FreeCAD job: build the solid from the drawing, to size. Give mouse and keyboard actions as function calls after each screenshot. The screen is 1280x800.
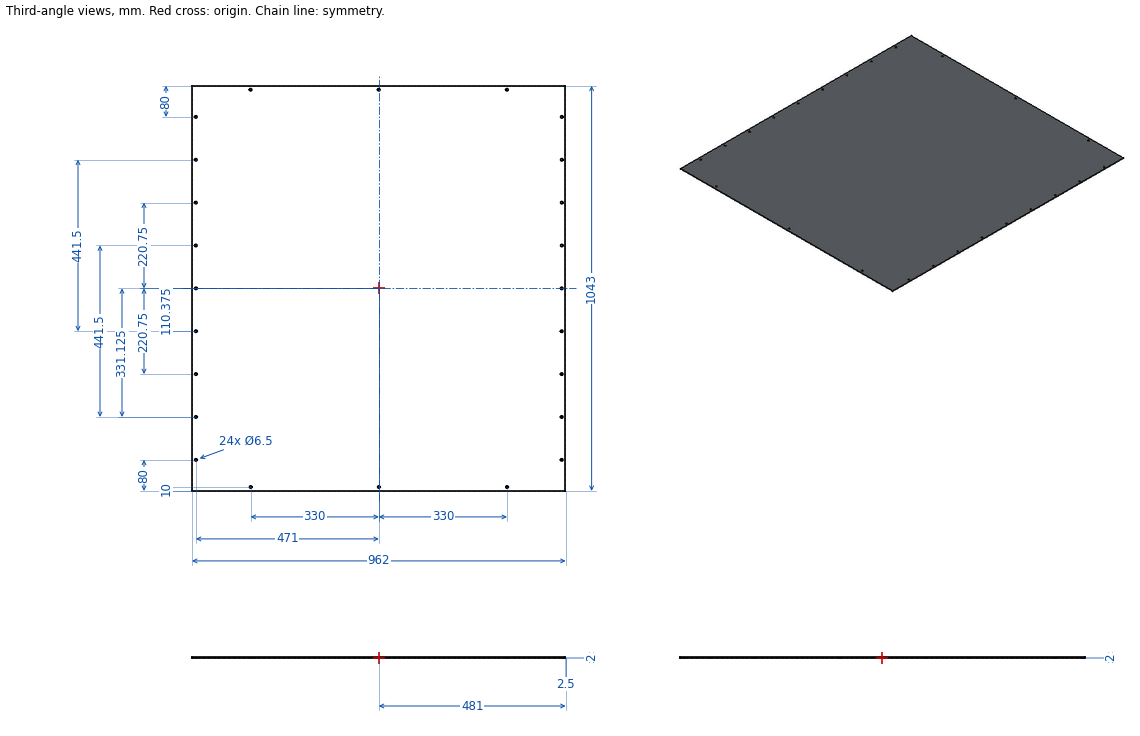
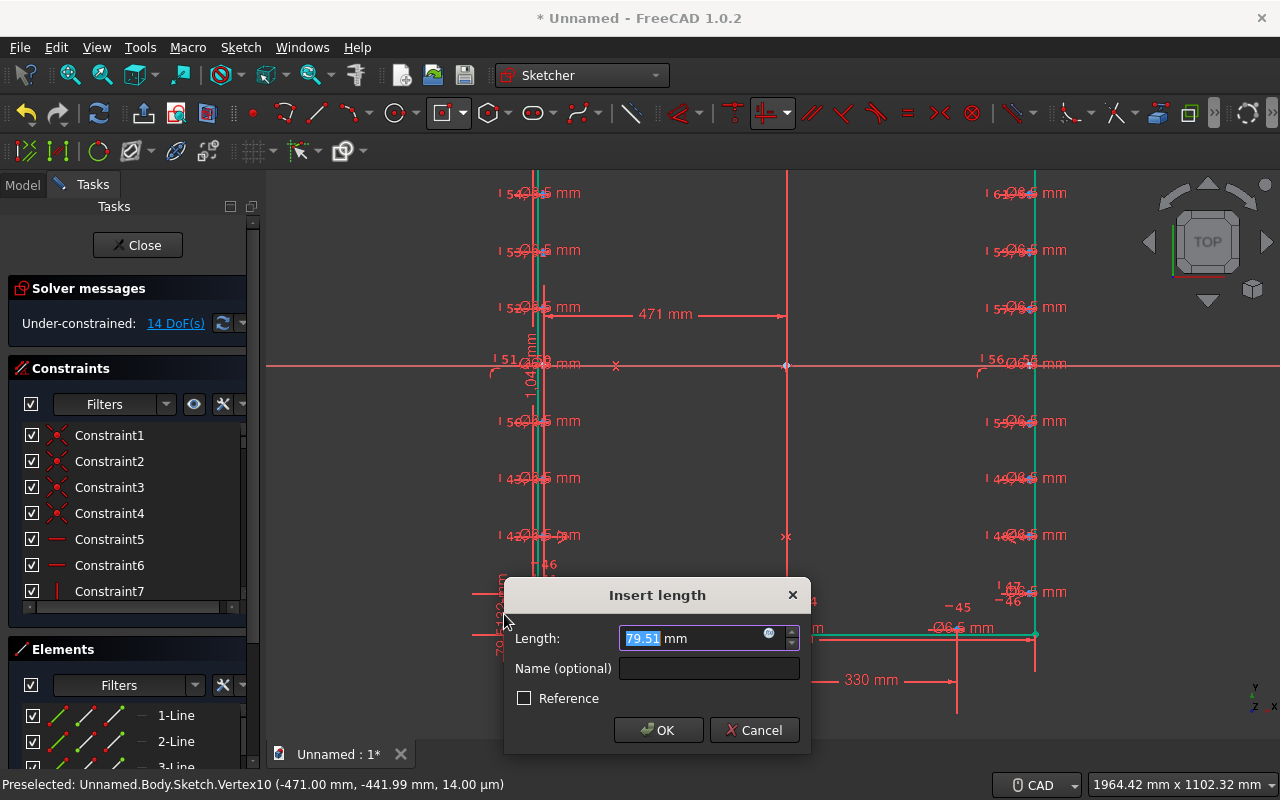
text(80)
key(Return)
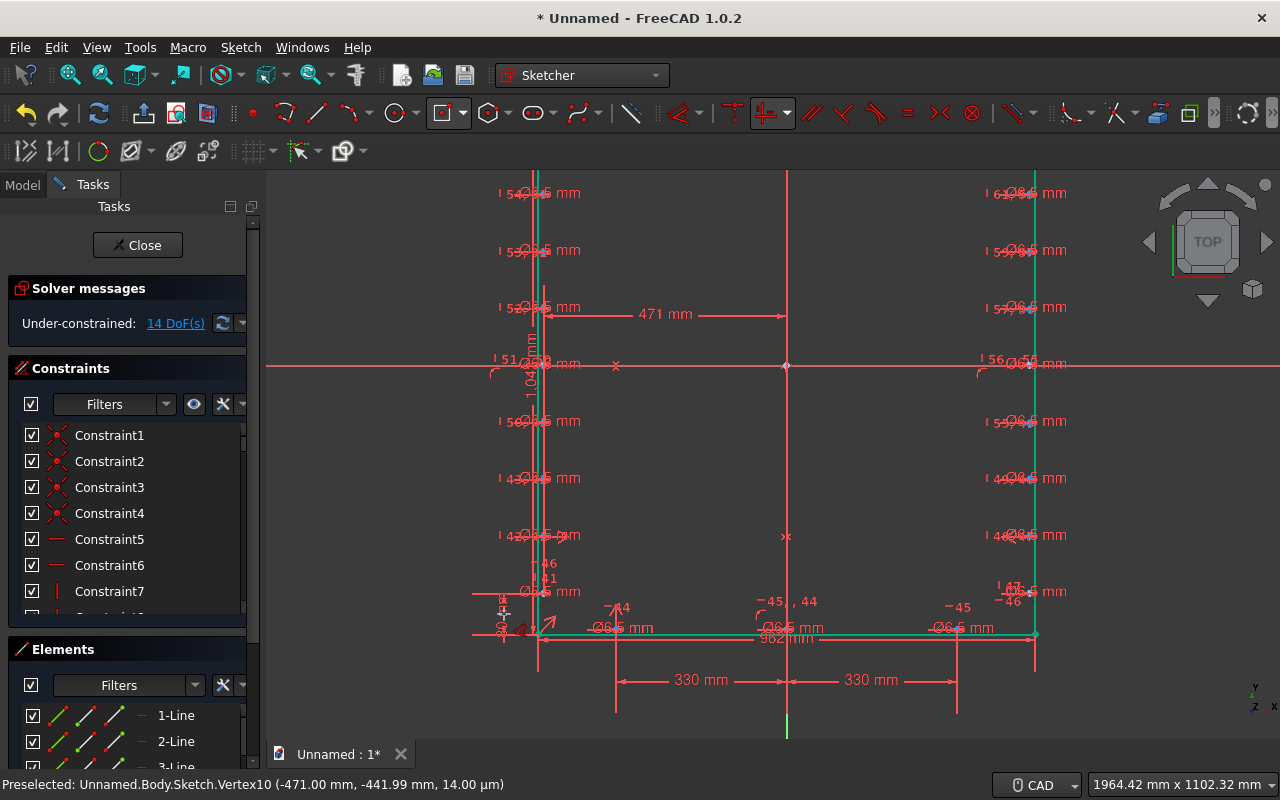
scroll(538, 635, up, 11)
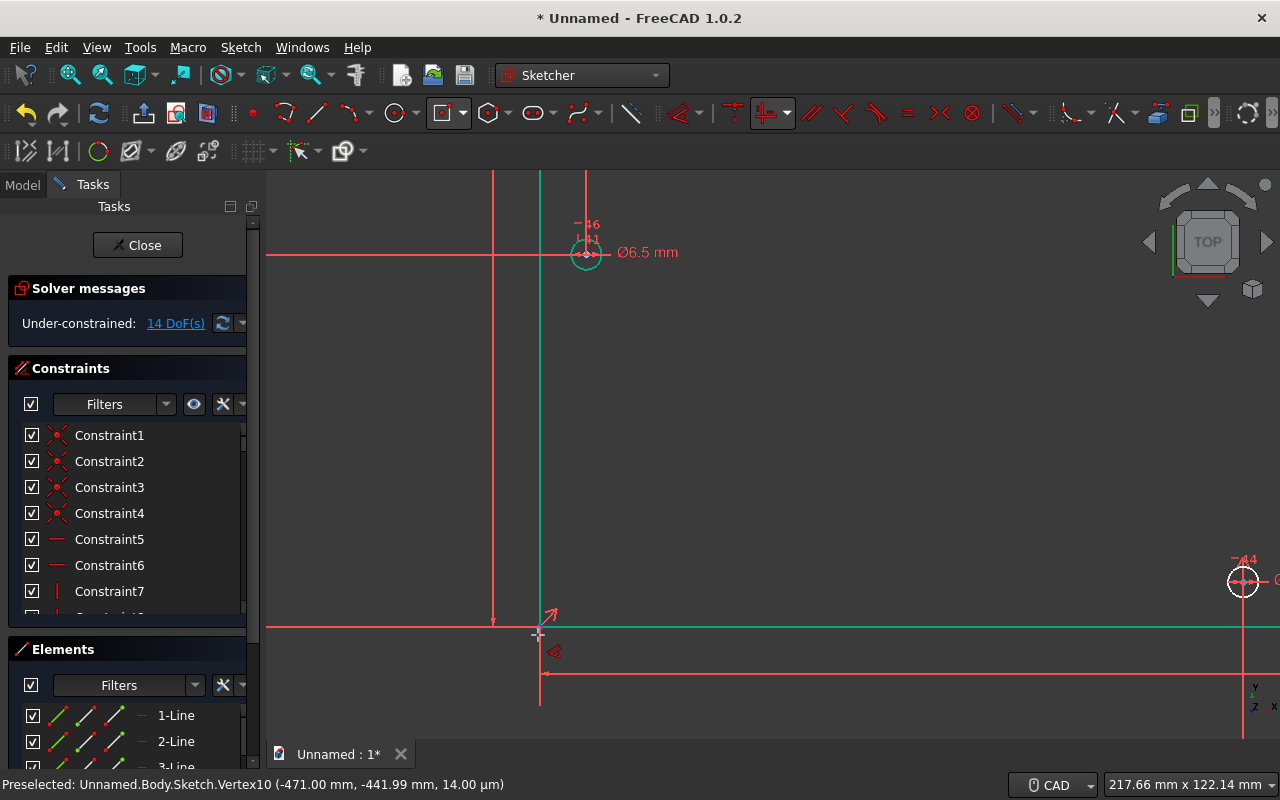
click(540, 627)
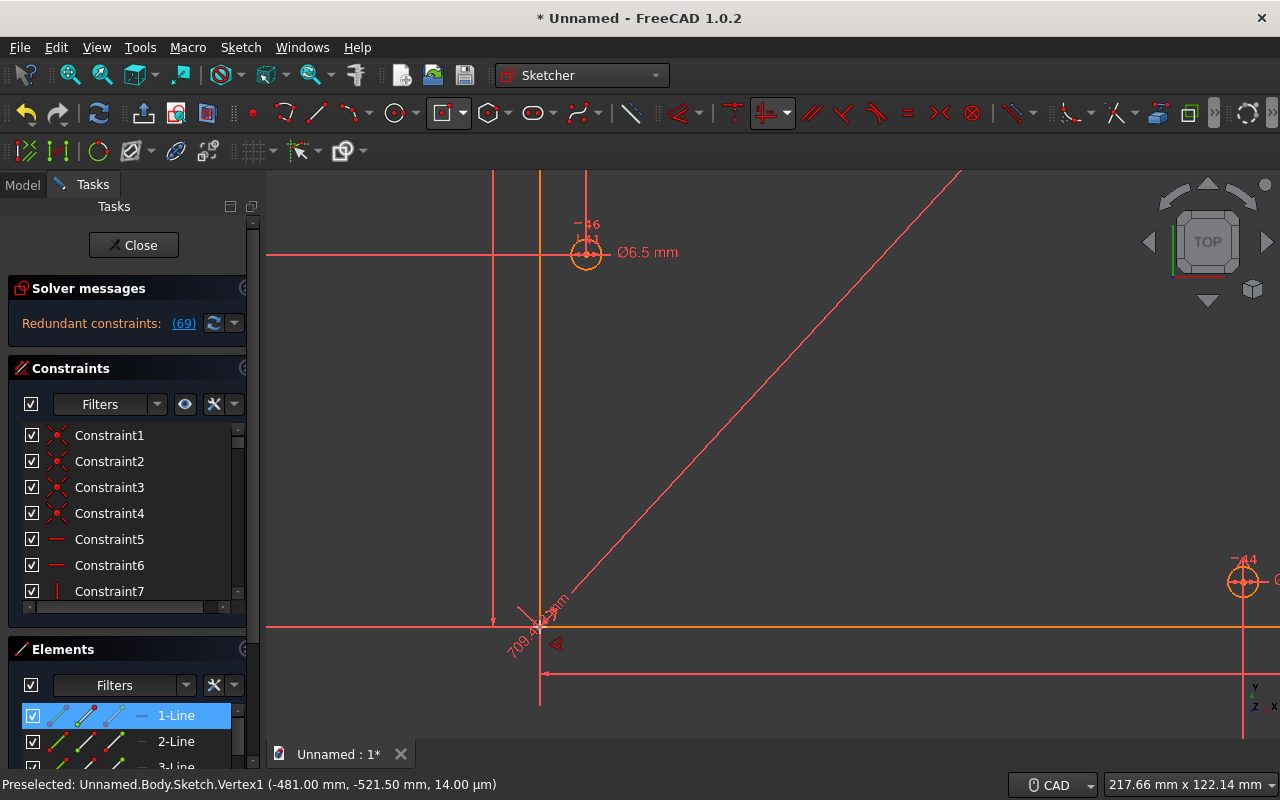
scroll(538, 636, down, 13)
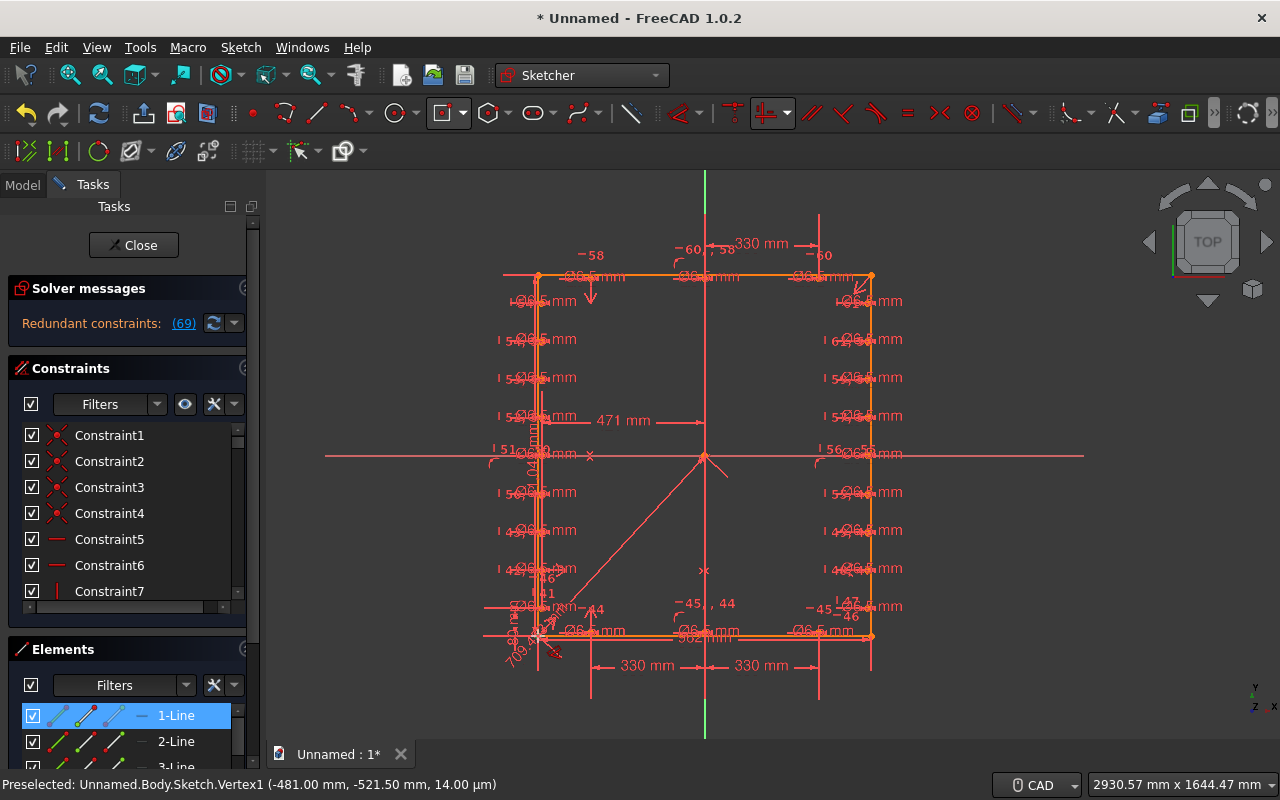
scroll(591, 633, up, 13)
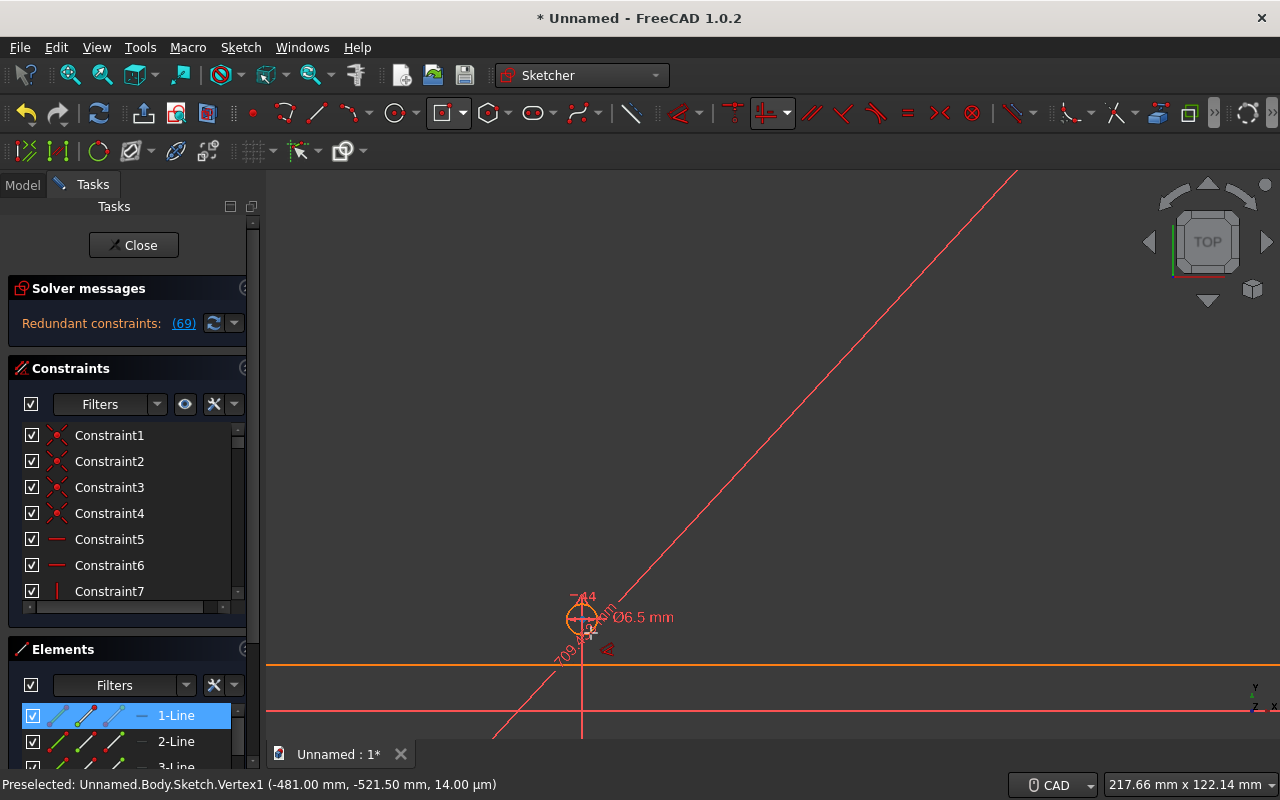
click(582, 619)
click(616, 642)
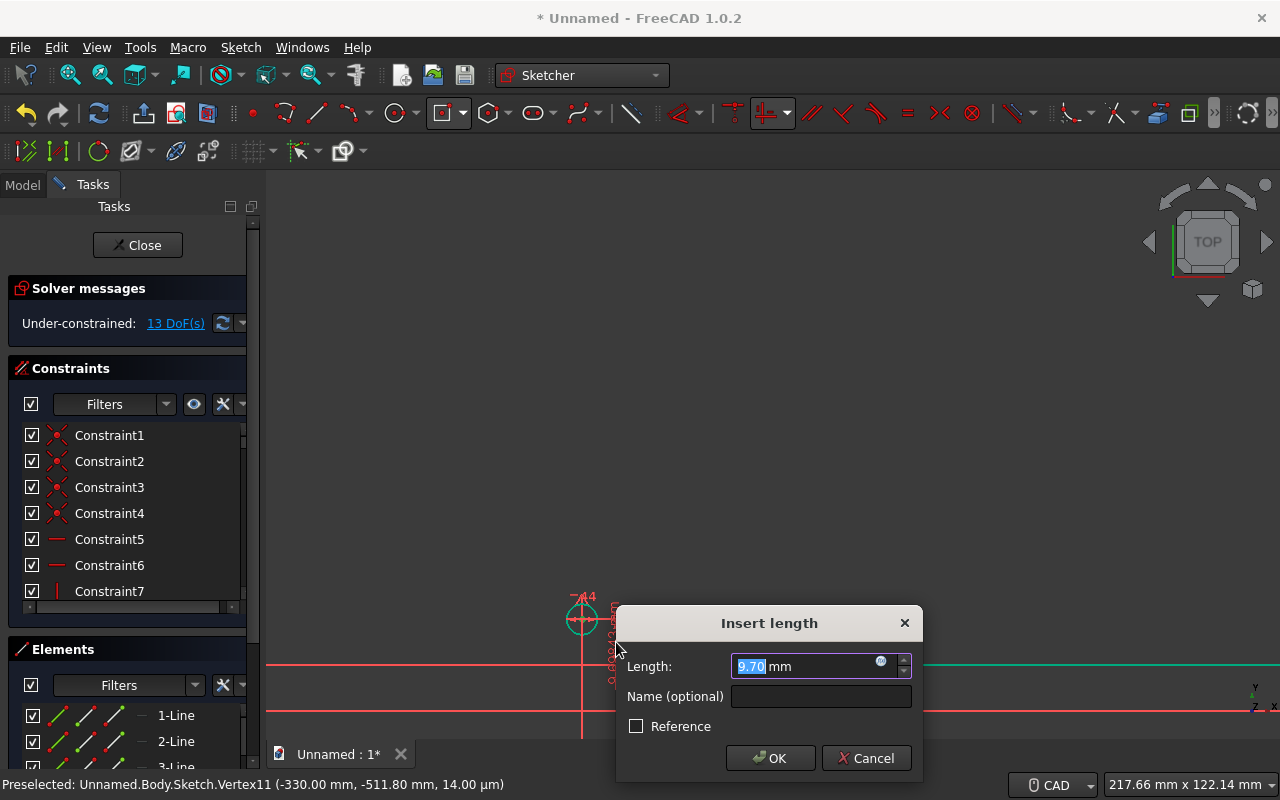
text(10)
key(Return)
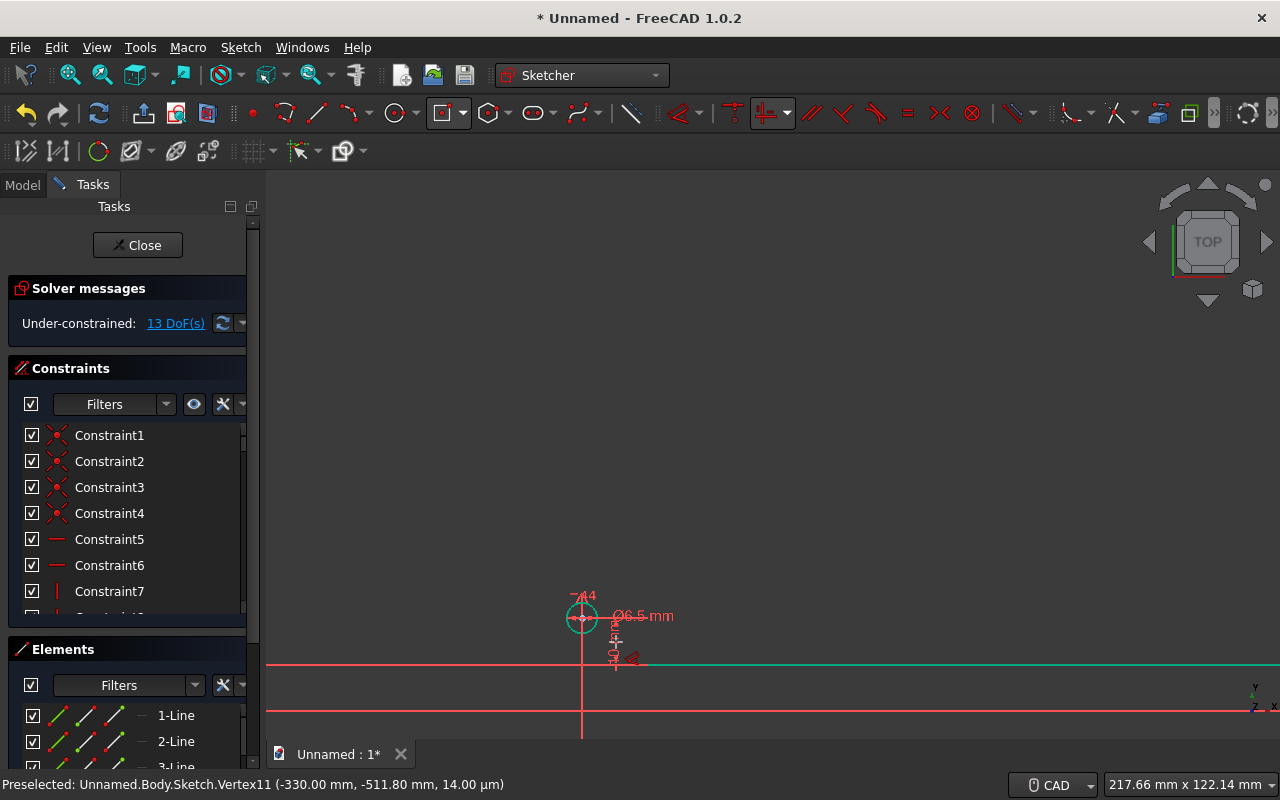
scroll(591, 633, down, 13)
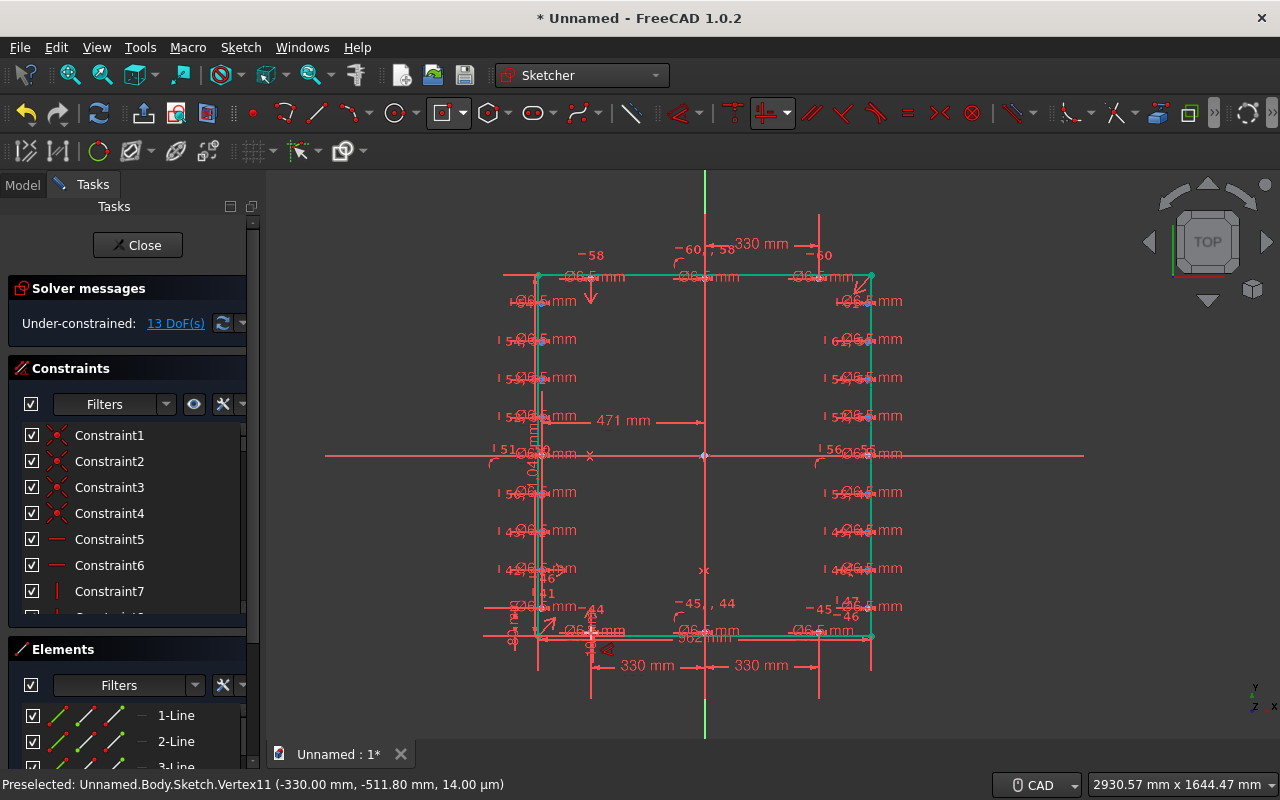
scroll(538, 275, up, 2)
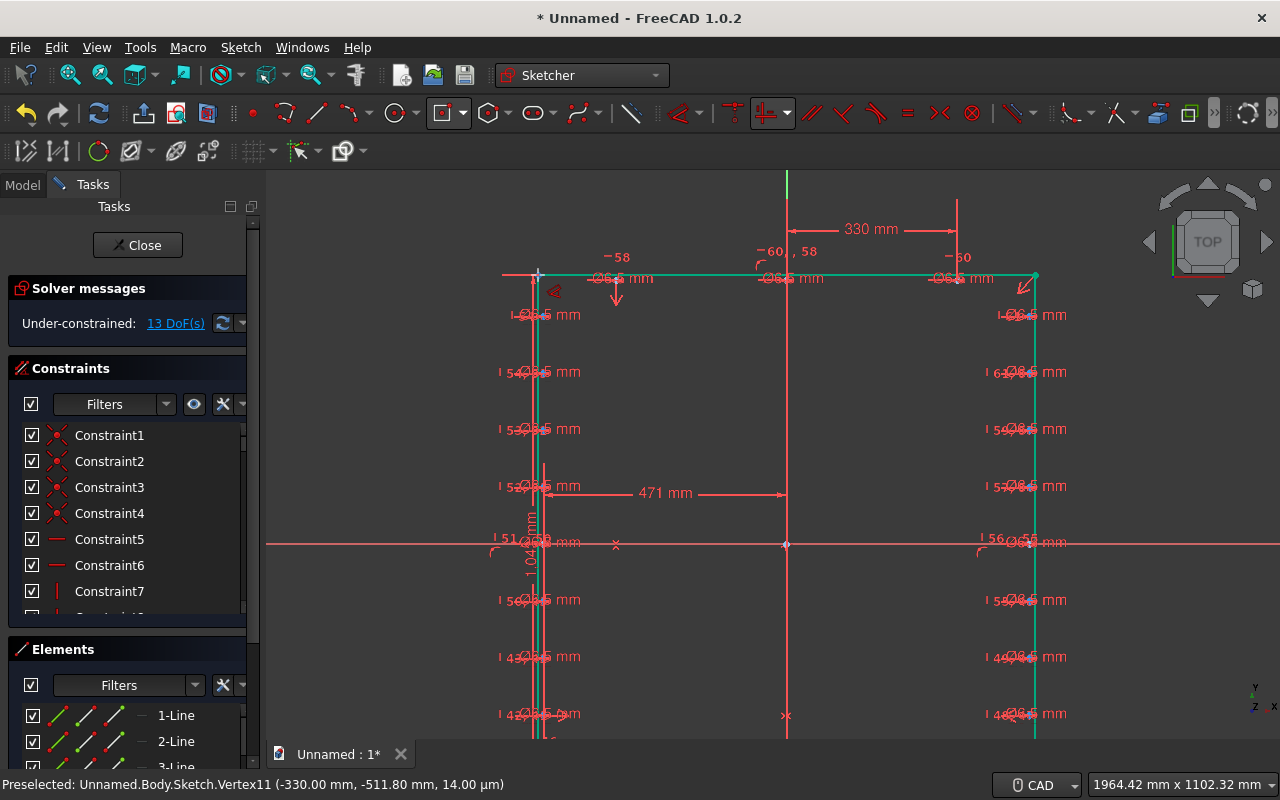
click(538, 275)